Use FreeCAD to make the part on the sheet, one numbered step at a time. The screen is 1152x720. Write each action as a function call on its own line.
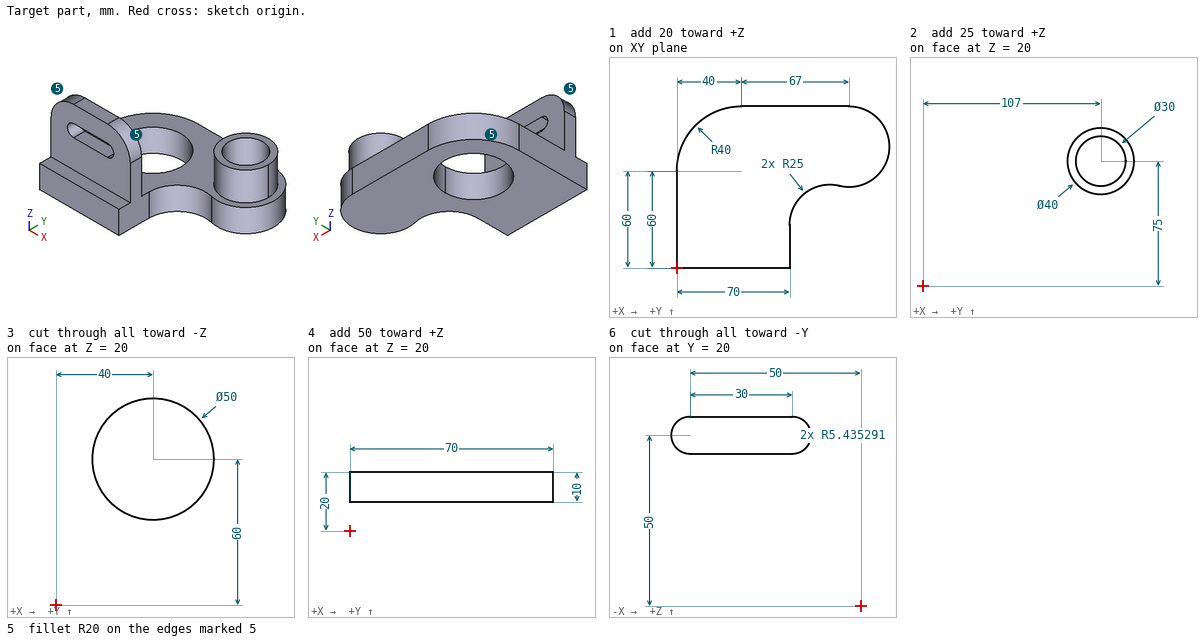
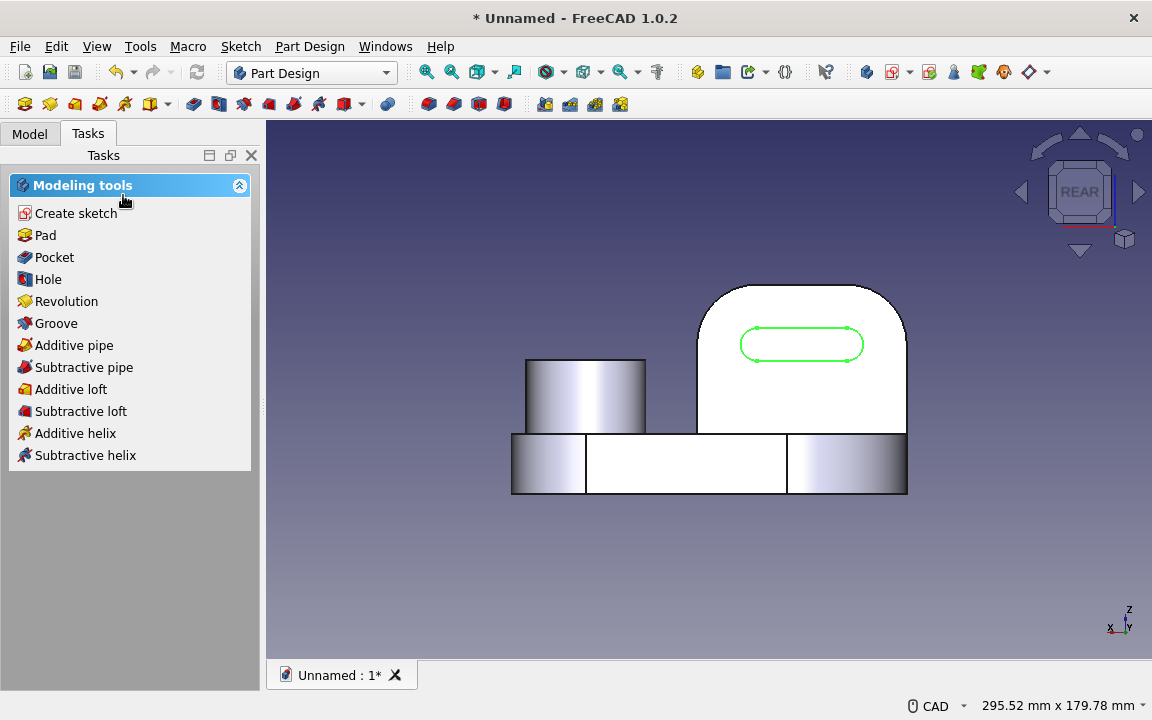
click(194, 104)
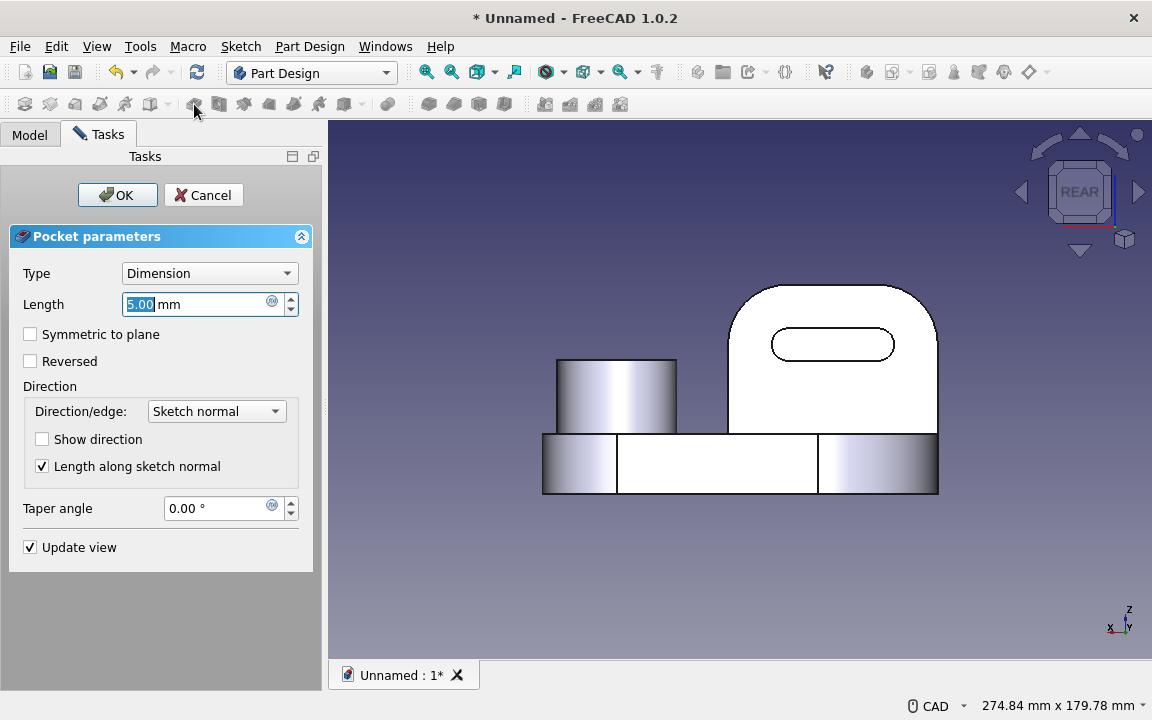
click(210, 274)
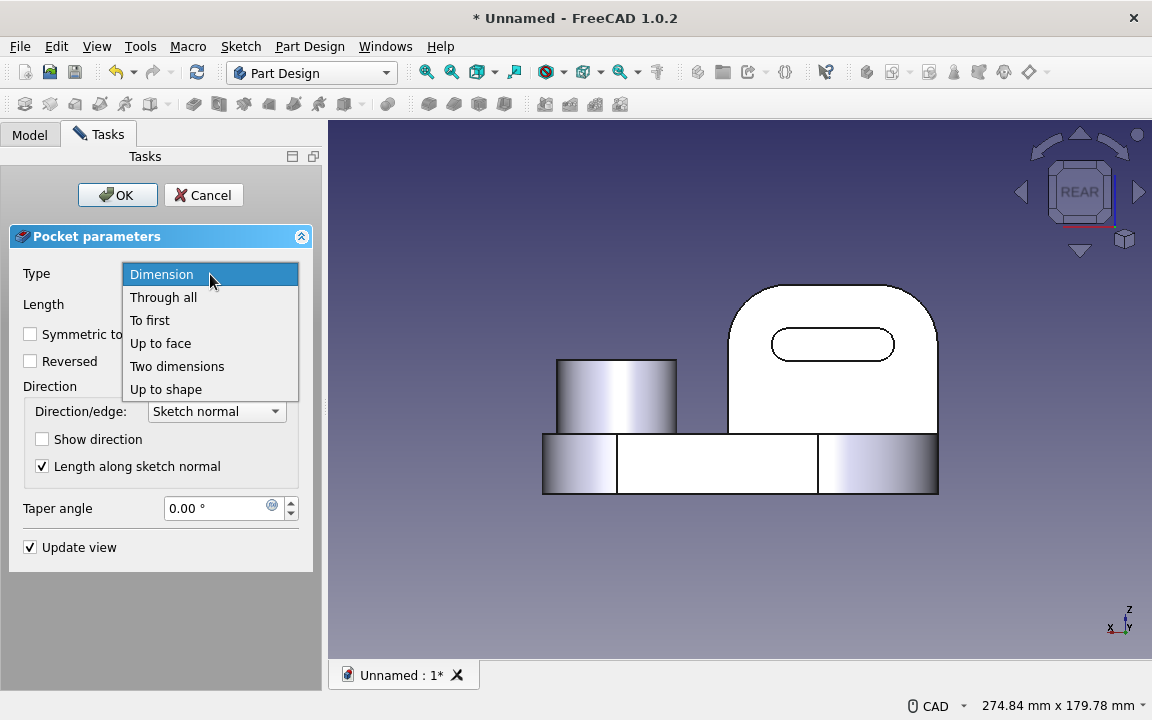
click(208, 298)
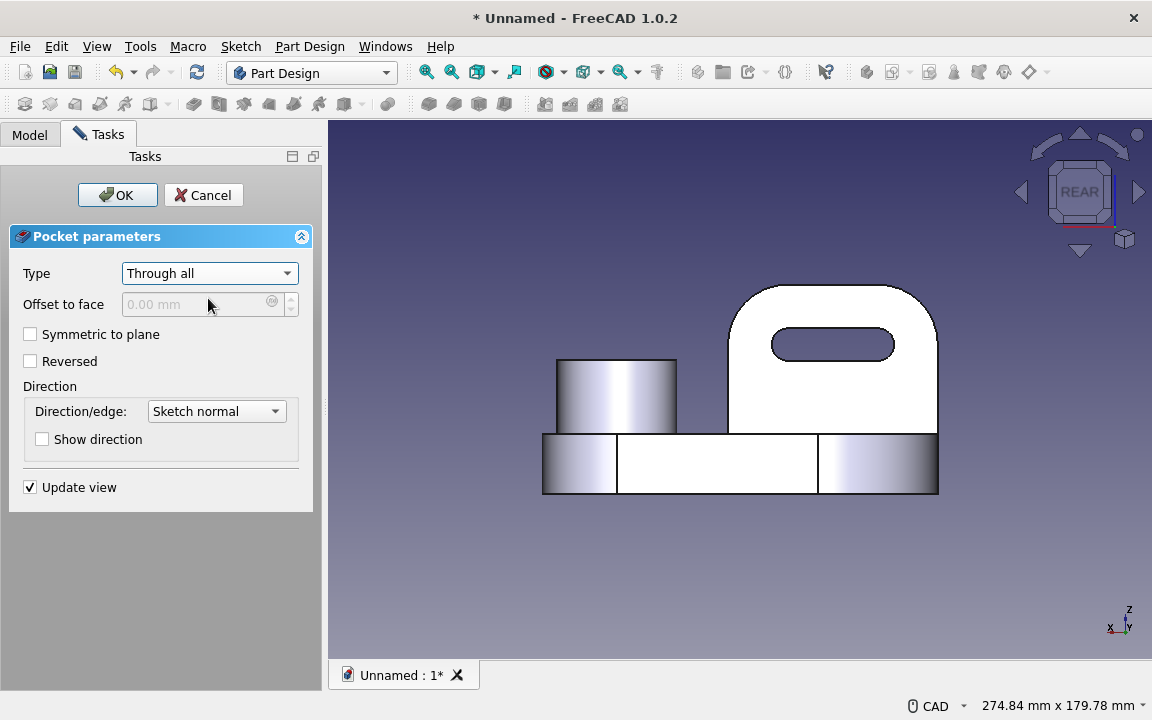
click(118, 195)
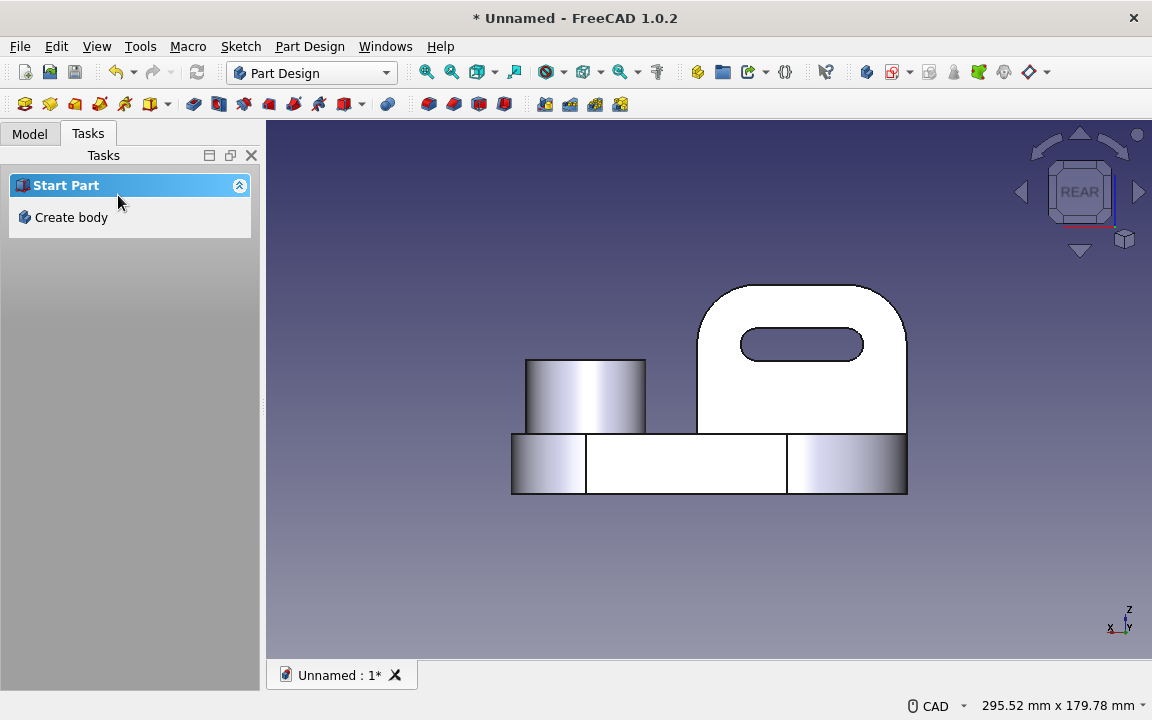
key(0)